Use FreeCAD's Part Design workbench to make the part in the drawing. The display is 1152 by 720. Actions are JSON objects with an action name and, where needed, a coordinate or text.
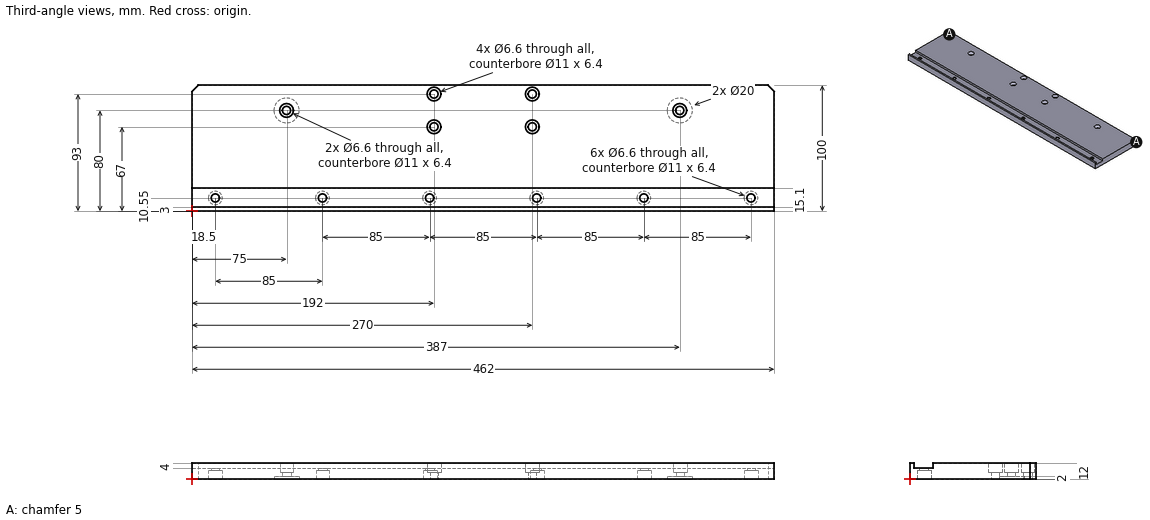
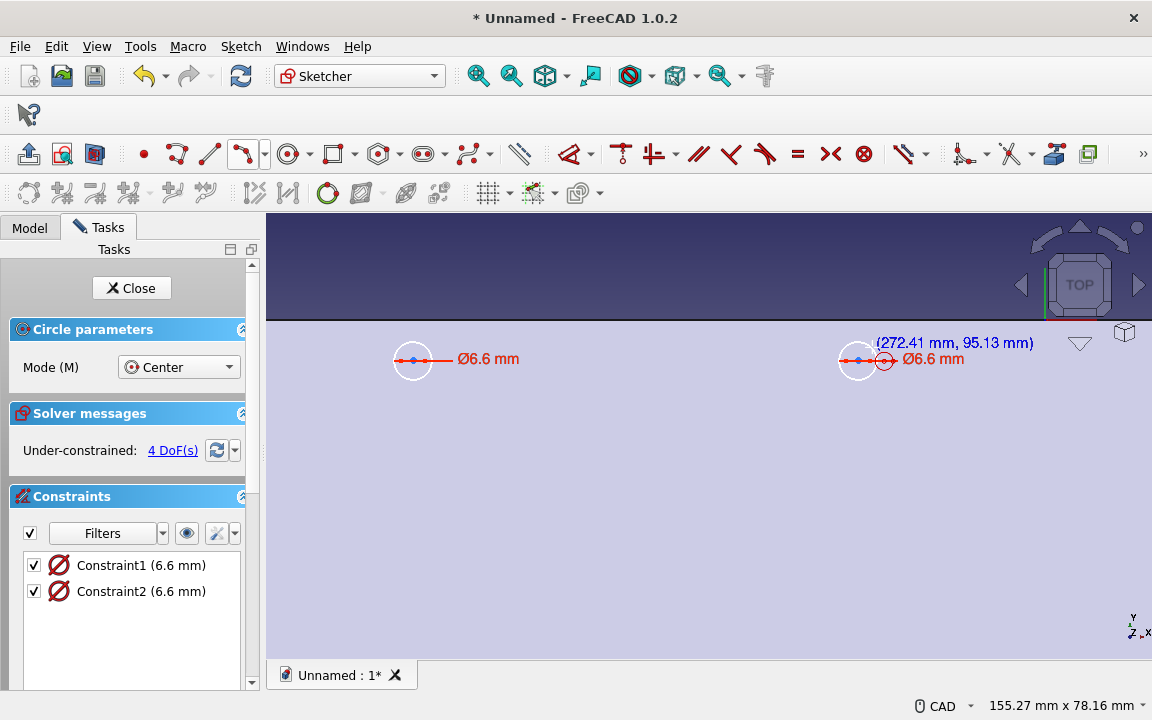
{"action": "left_click", "coordinate": [413, 509]}
{"action": "mouse_move", "coordinate": [426, 495]}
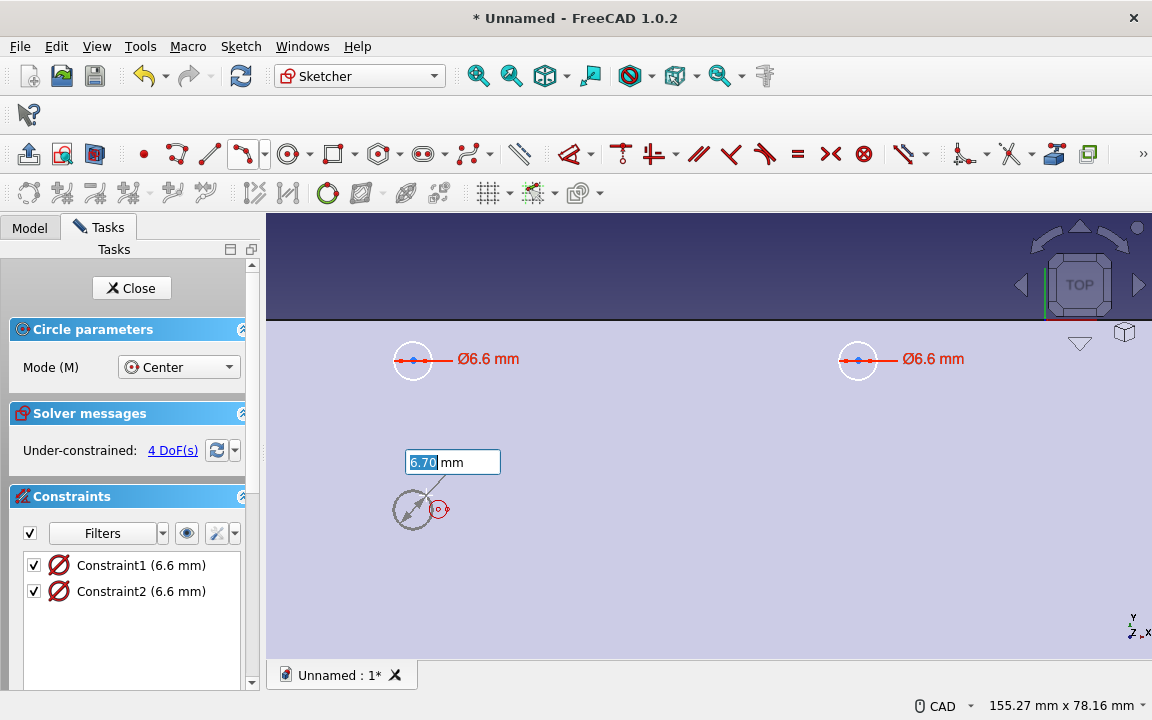
{"action": "type", "text": "6.6"}
{"action": "key", "text": "Return"}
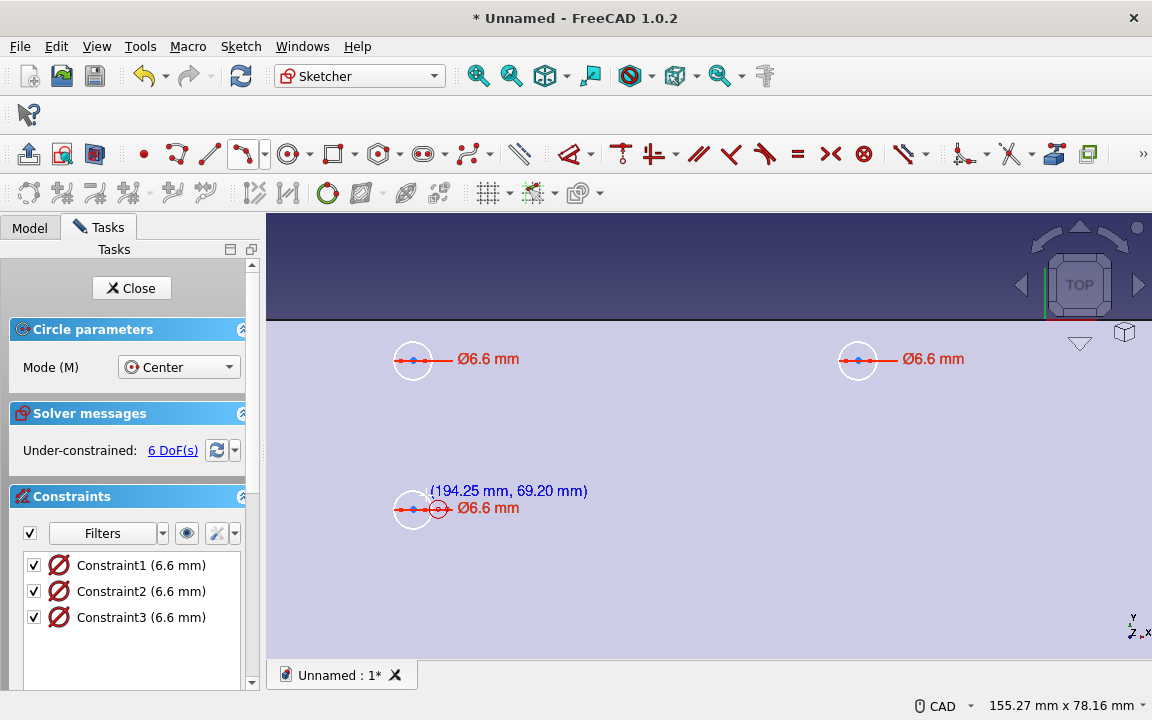
{"action": "left_click", "coordinate": [858, 509]}
{"action": "mouse_move", "coordinate": [872, 495]}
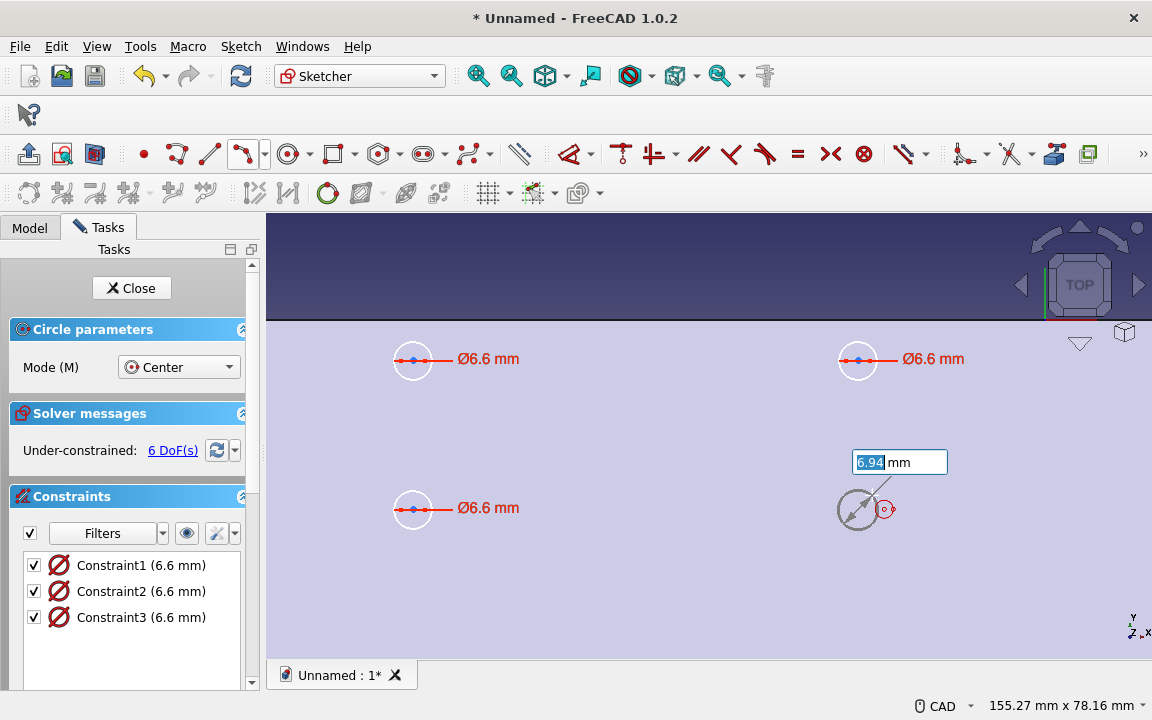
{"action": "type", "text": "6.6"}
{"action": "key", "text": "Return"}
{"action": "key", "text": "Escape"}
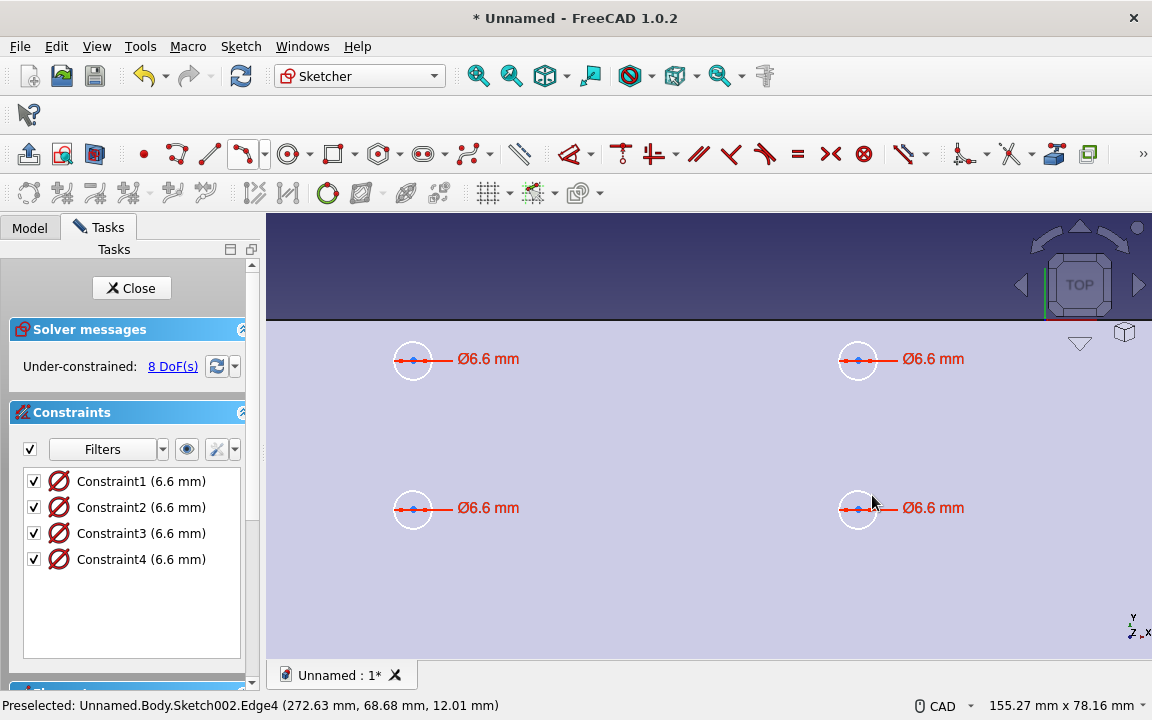
{"action": "left_click", "coordinate": [413, 361]}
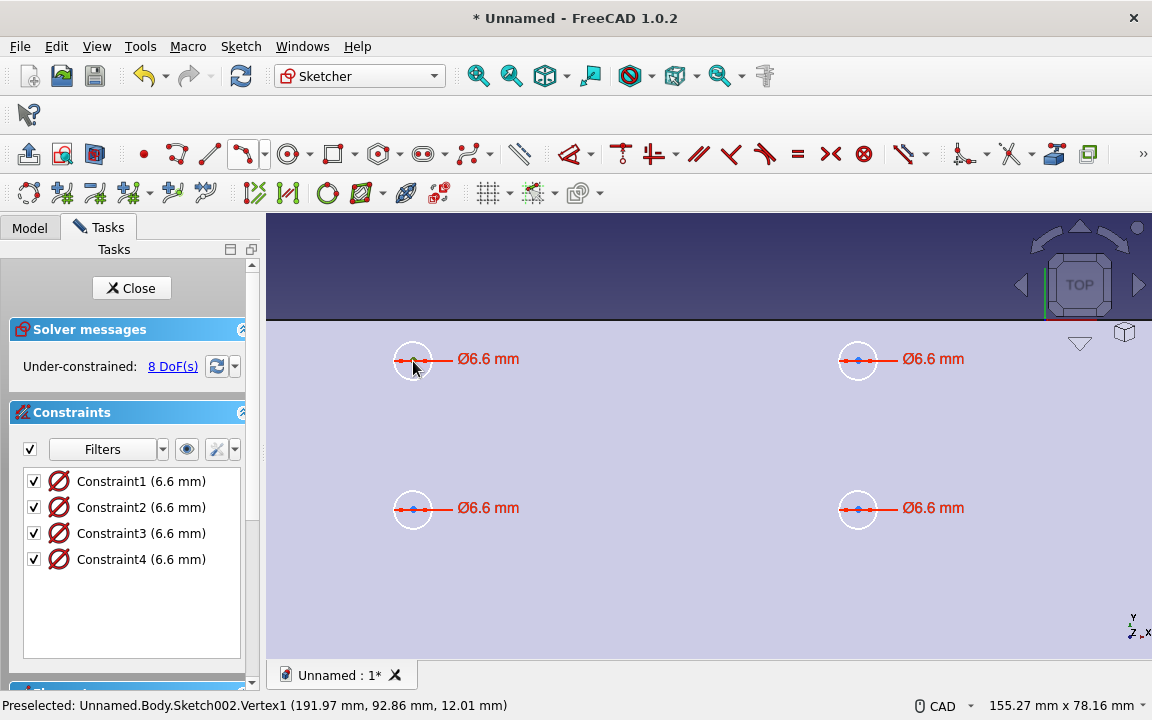
{"action": "left_click", "coordinate": [858, 361]}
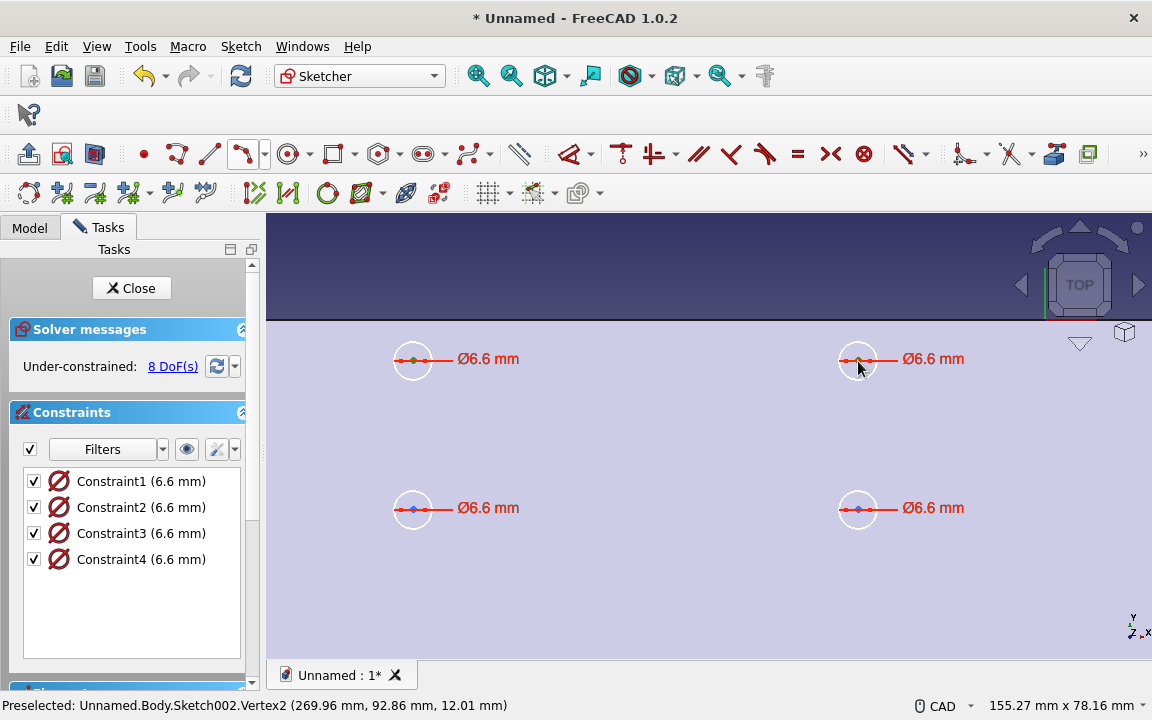
{"action": "left_click", "coordinate": [676, 154]}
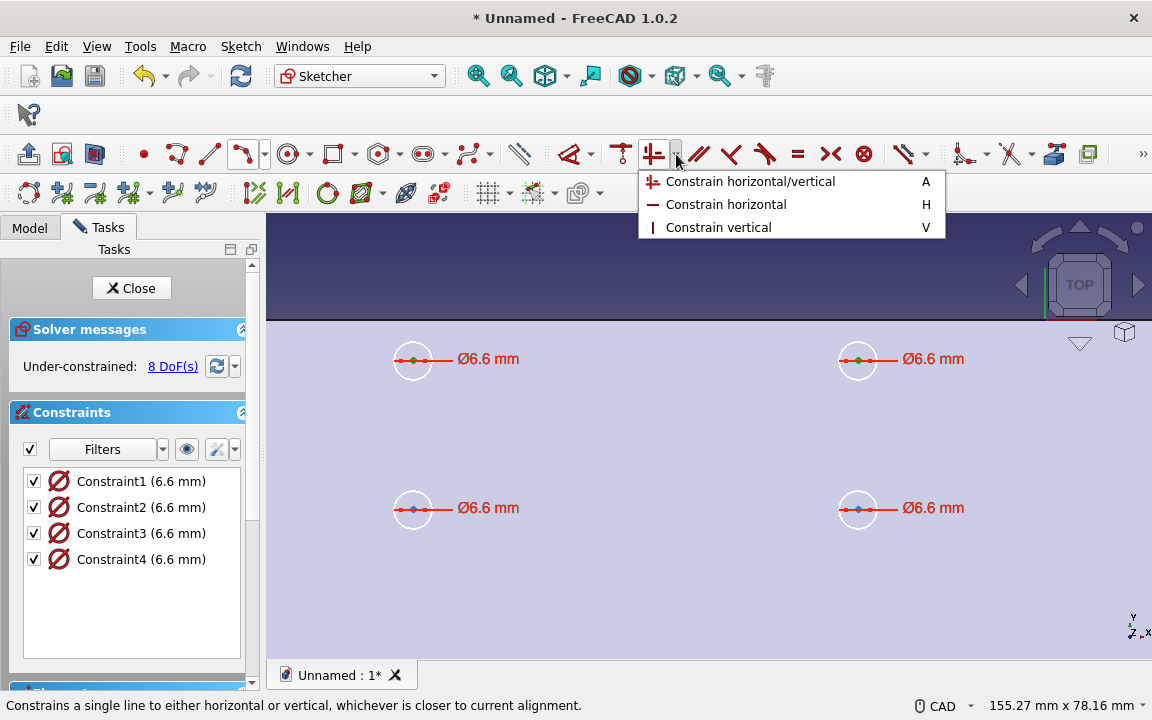
{"action": "left_click", "coordinate": [792, 204]}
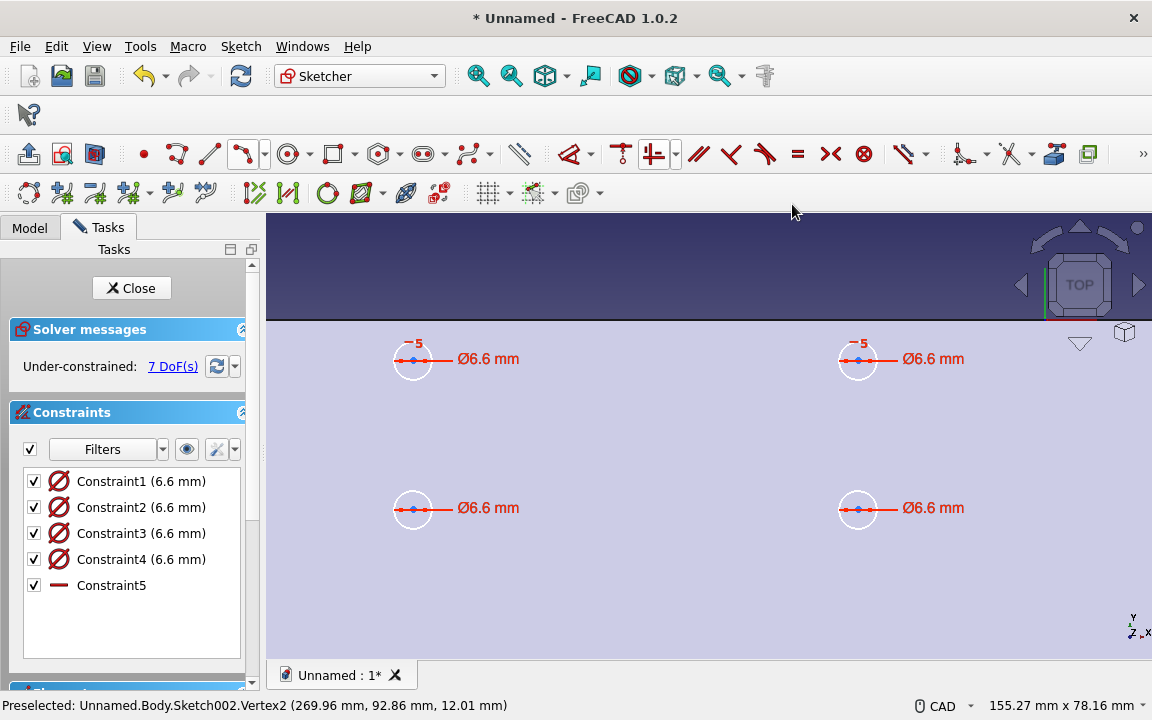
{"action": "left_click", "coordinate": [413, 361]}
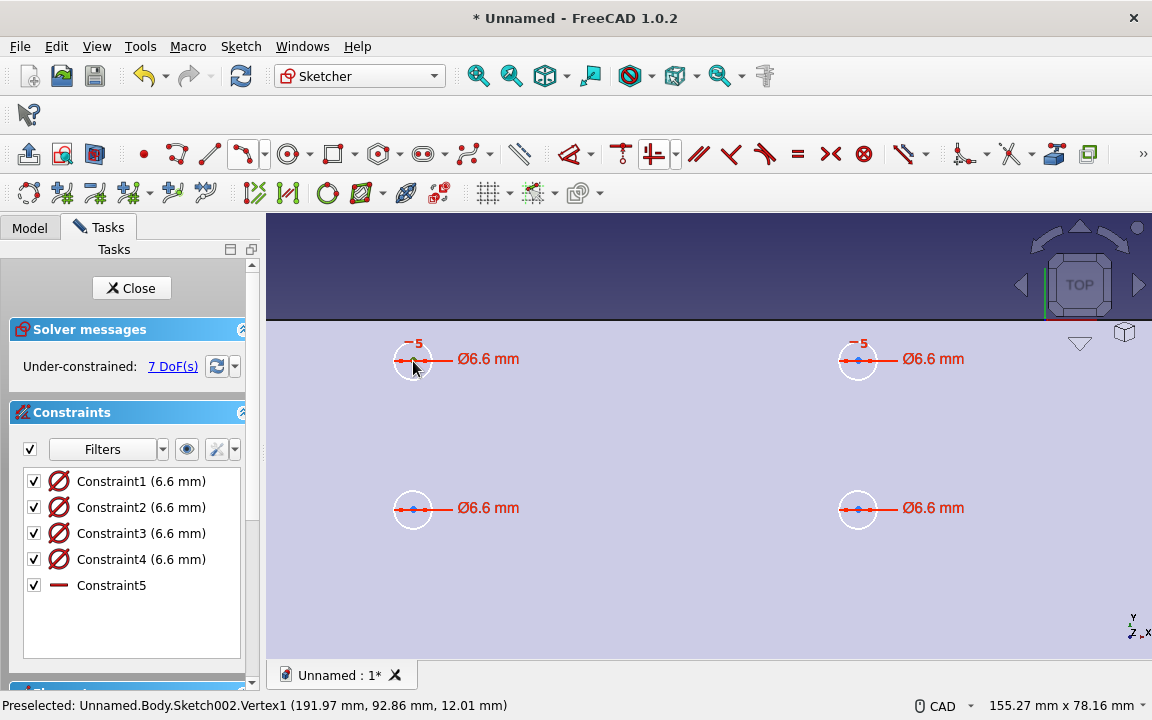
{"action": "left_click", "coordinate": [413, 510]}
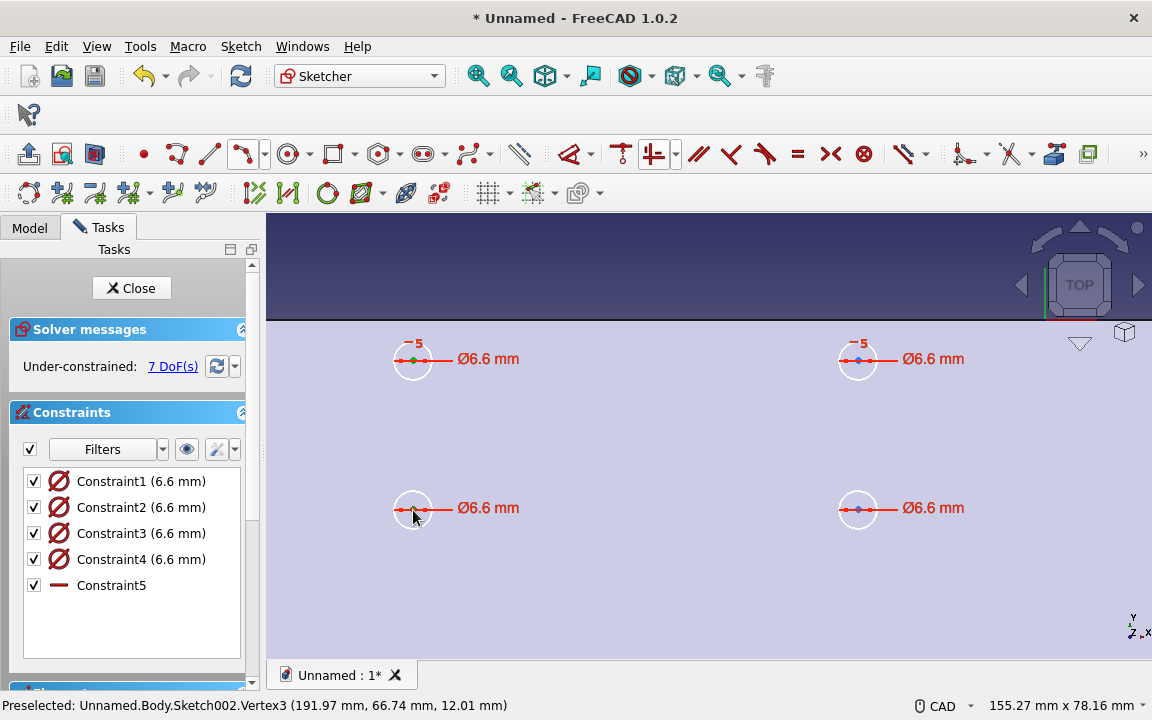
{"action": "left_click", "coordinate": [676, 154]}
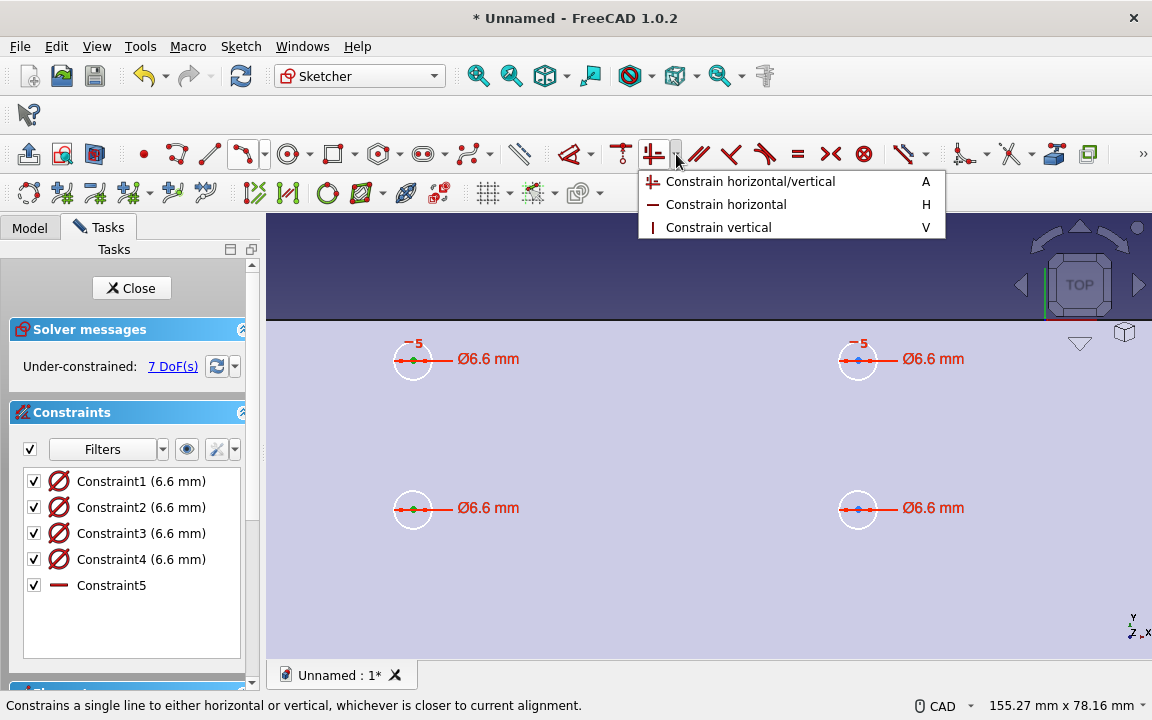
{"action": "left_click", "coordinate": [792, 228]}